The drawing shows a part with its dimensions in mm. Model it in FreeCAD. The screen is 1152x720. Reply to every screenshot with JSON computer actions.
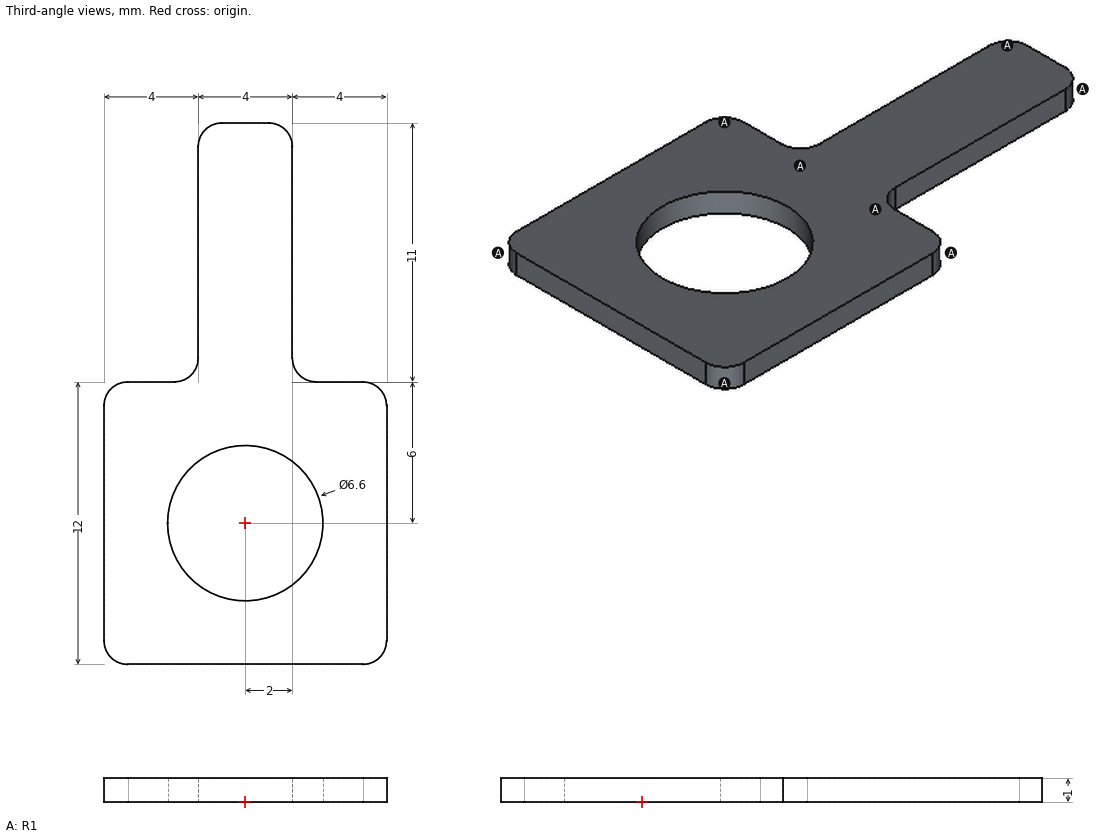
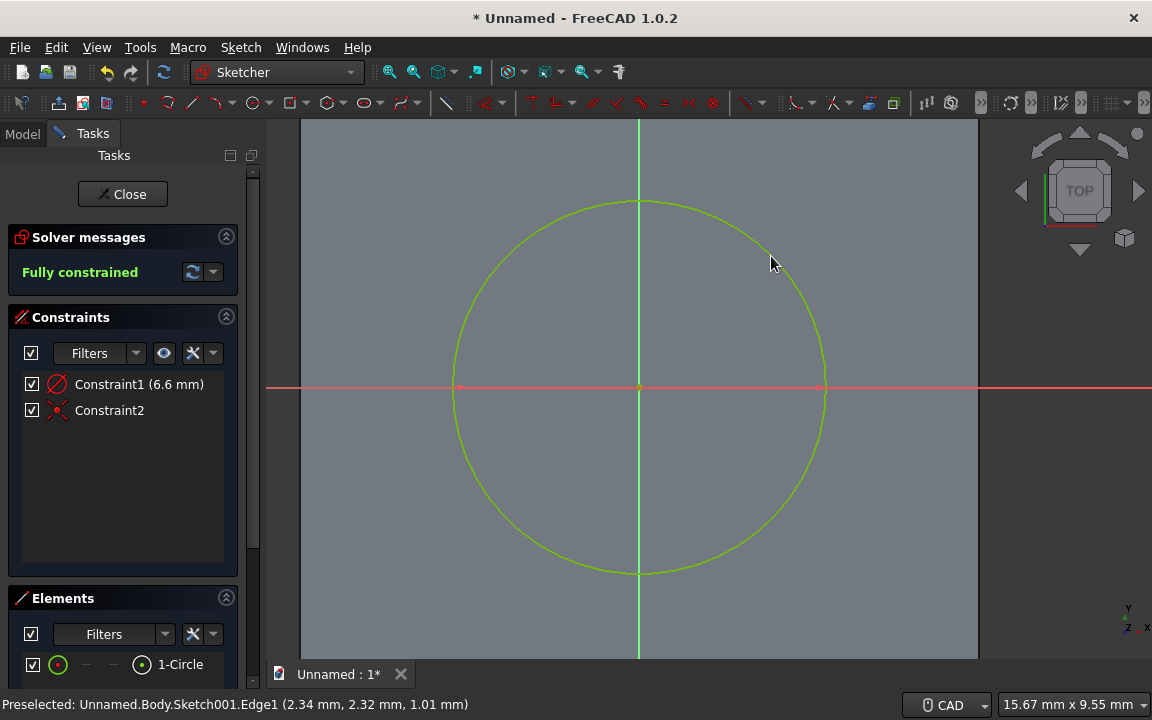
{"action": "left_click", "coordinate": [123, 194]}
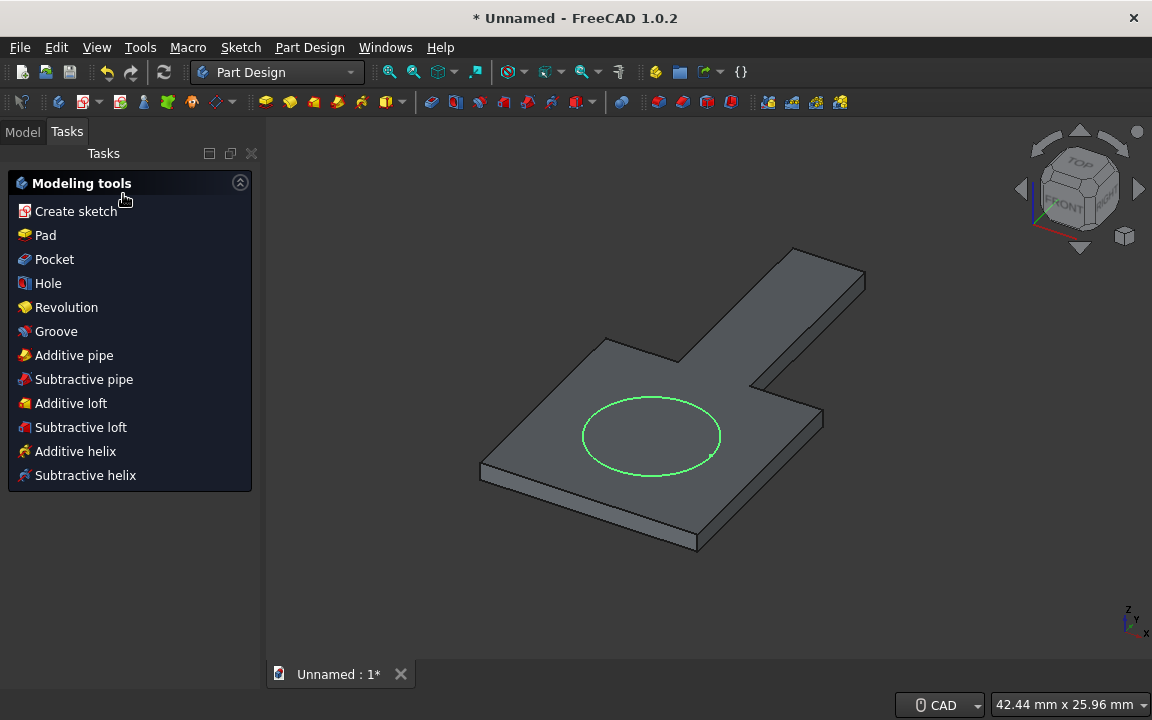
{"action": "left_click", "coordinate": [432, 102]}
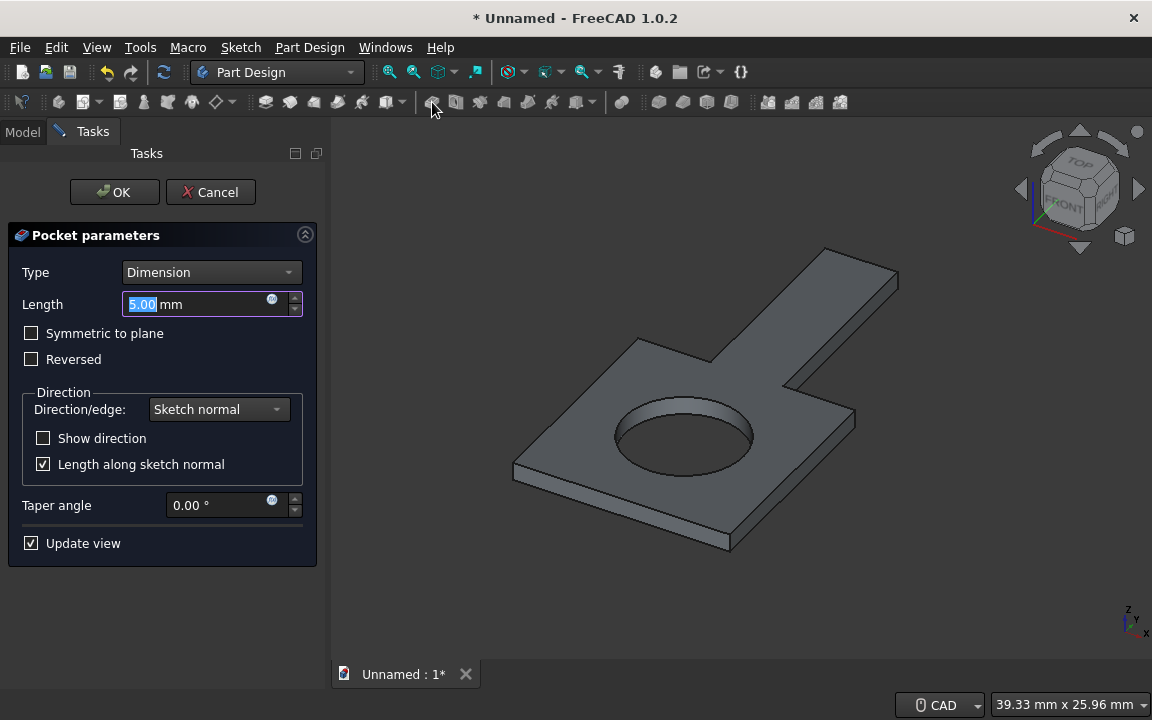
{"action": "left_click", "coordinate": [212, 272]}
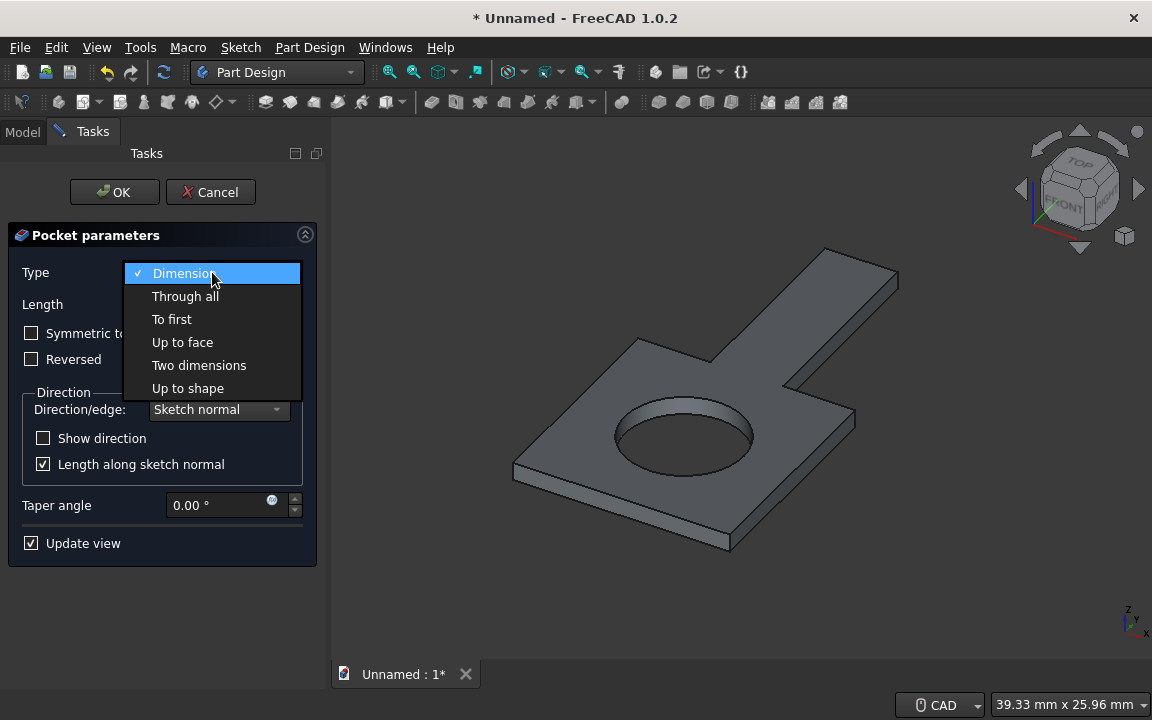
{"action": "left_click", "coordinate": [212, 296]}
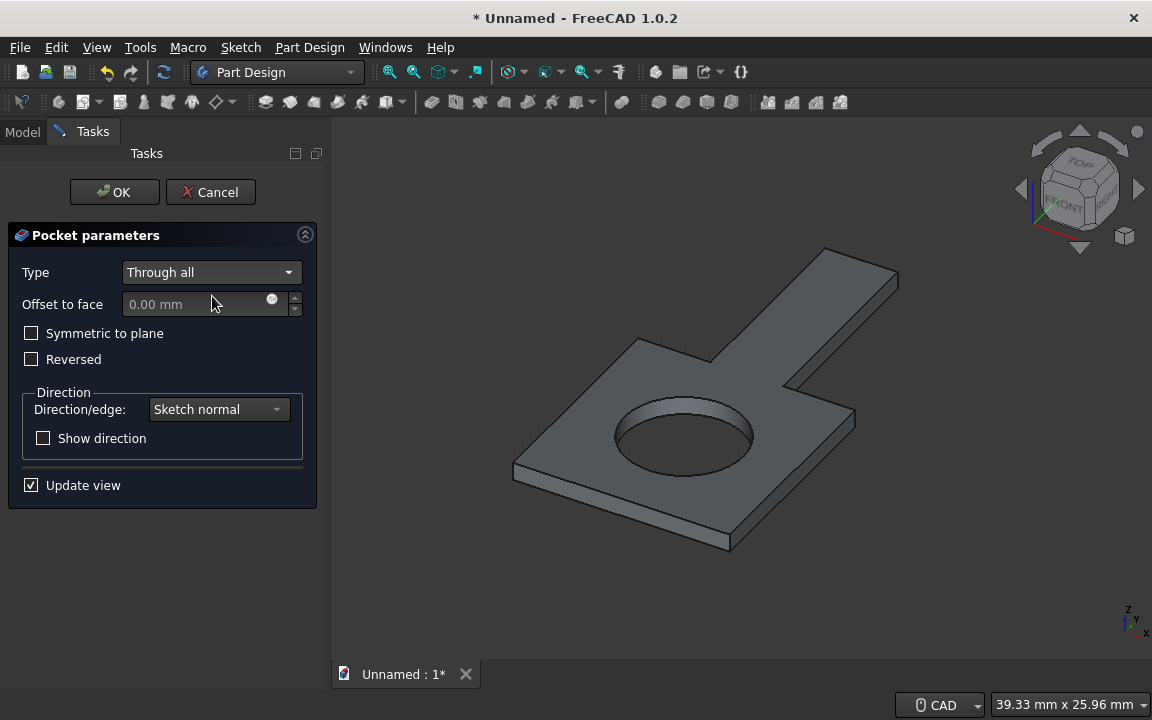
{"action": "left_click", "coordinate": [115, 192]}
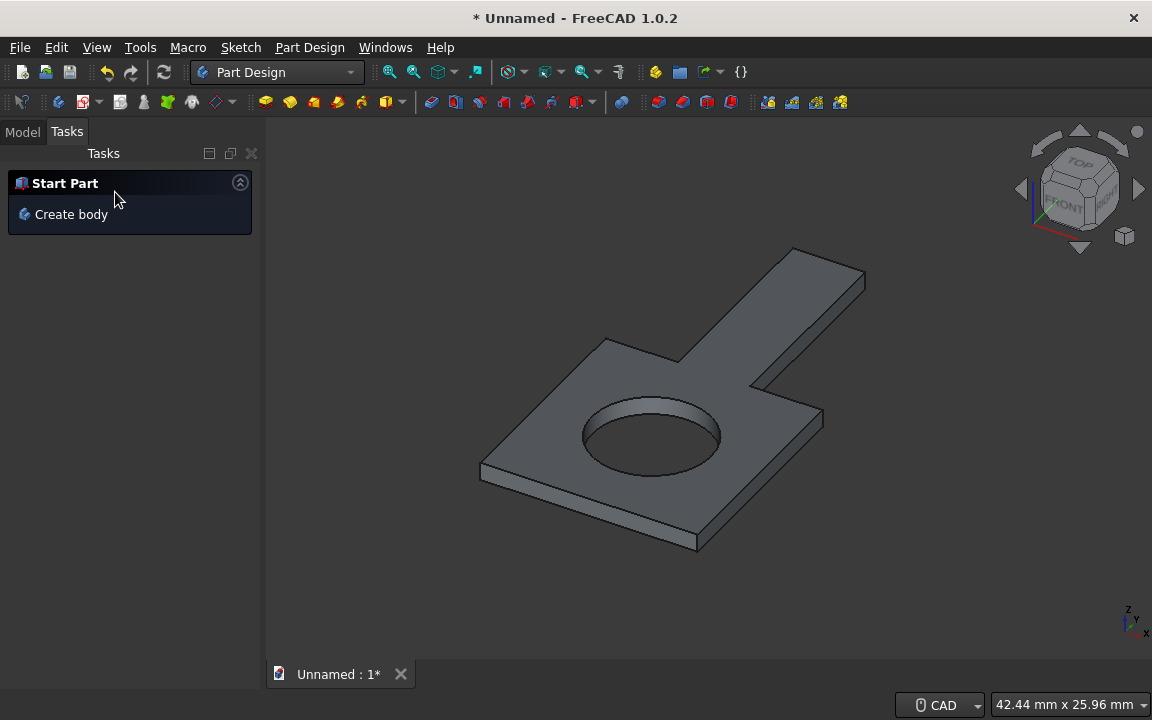
{"action": "left_click", "coordinate": [697, 542]}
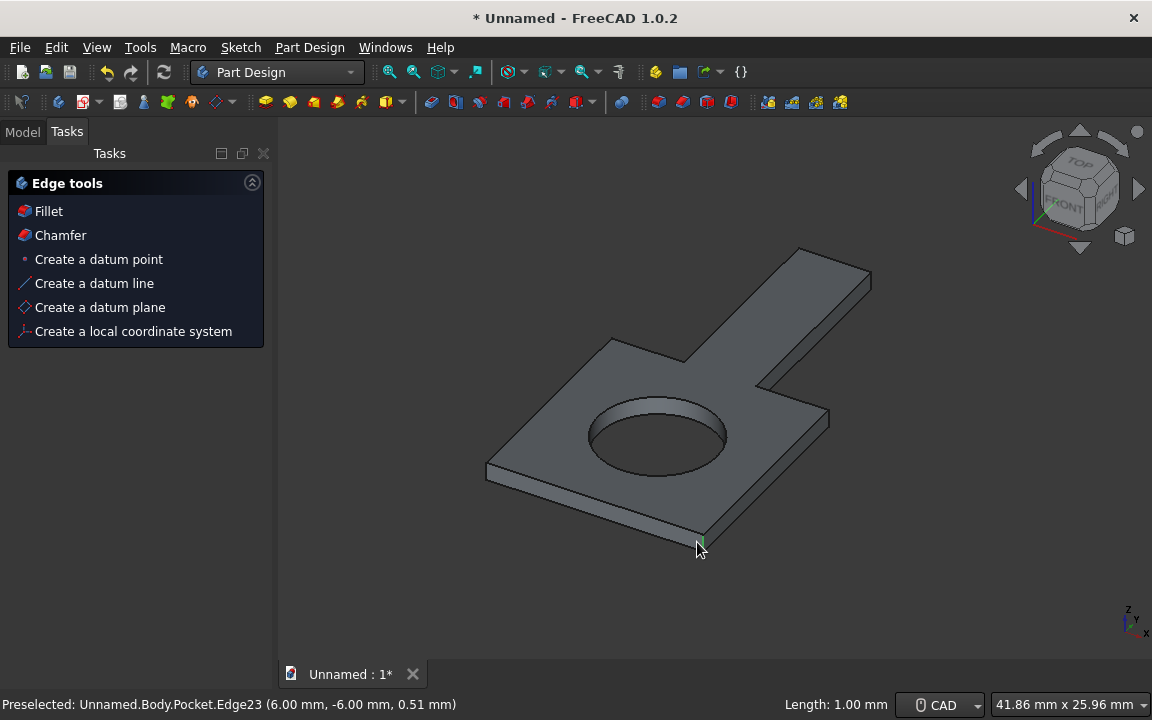
{"action": "scroll", "coordinate": [486, 470], "scroll_direction": "up", "scroll_amount": 4}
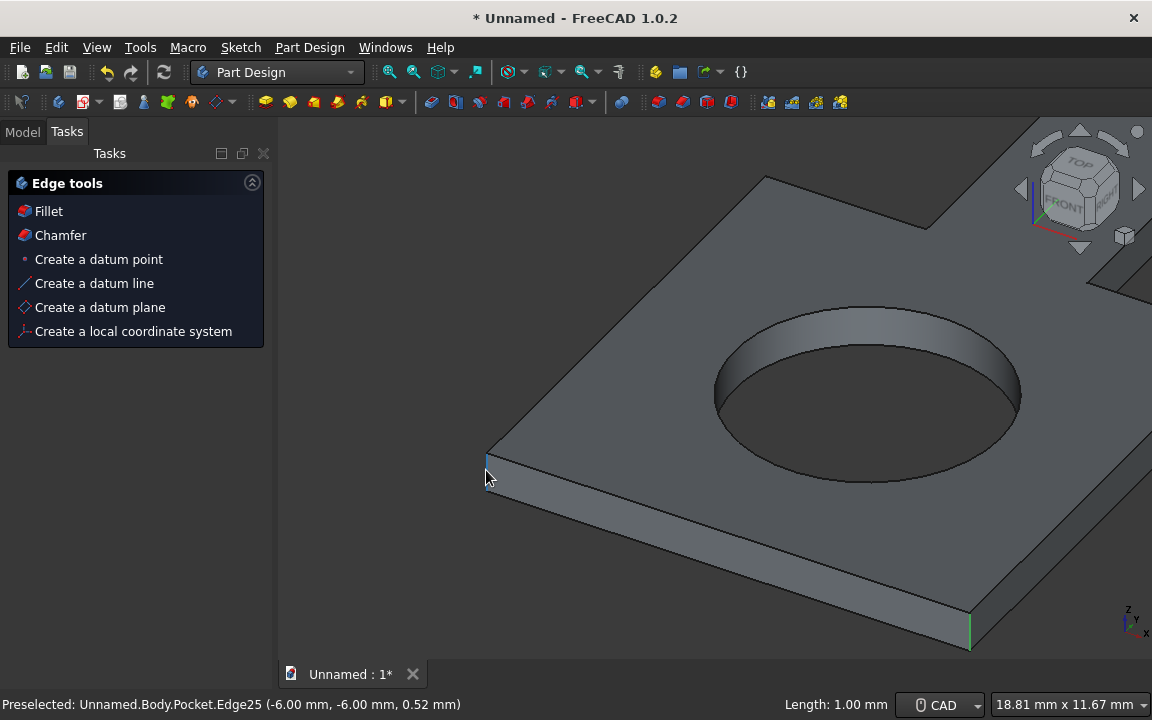
{"action": "left_click", "coordinate": [390, 72]}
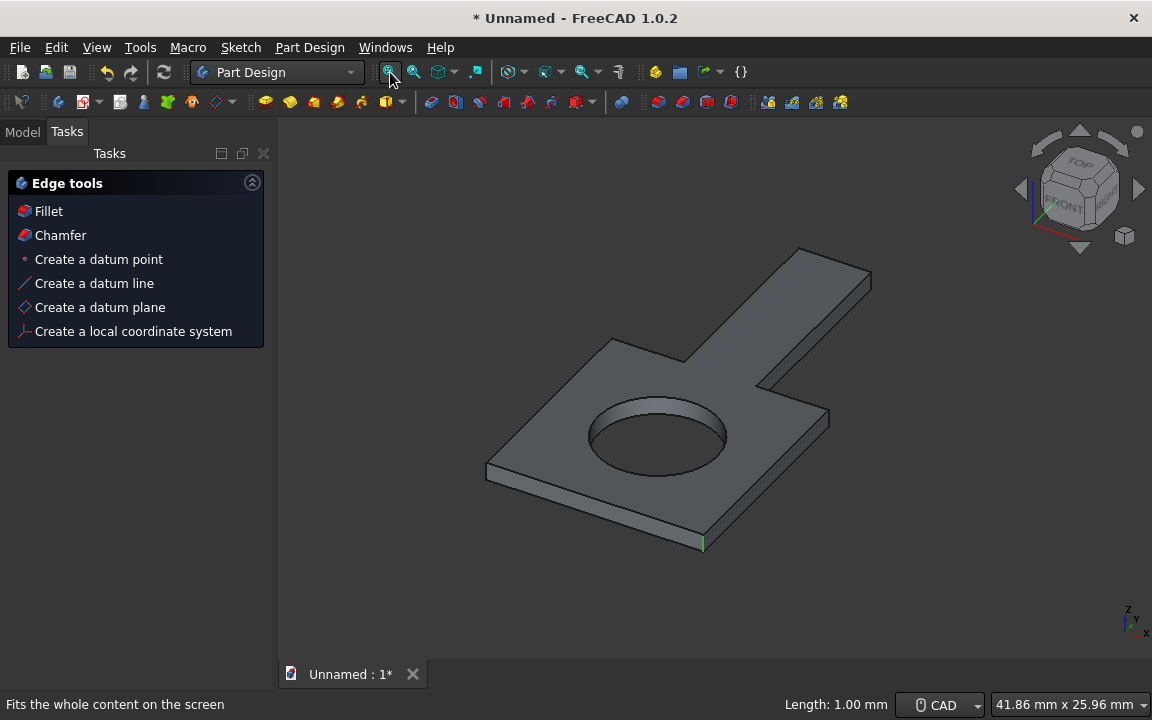
{"action": "key", "text": "0"}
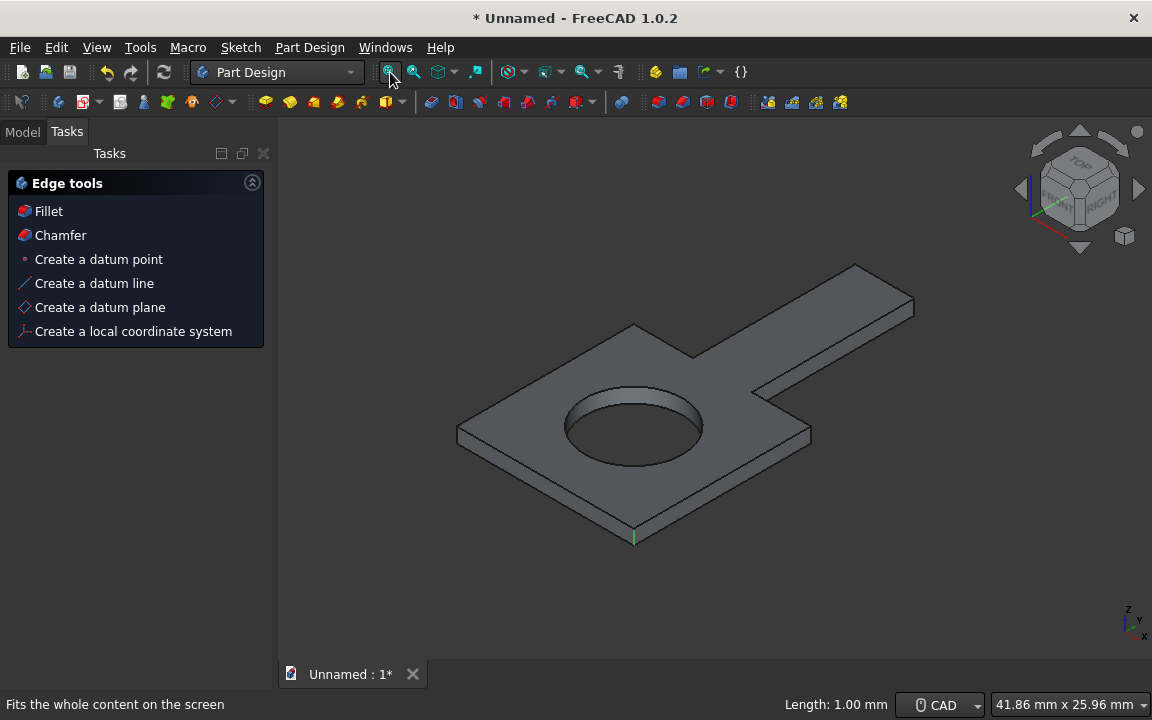
{"action": "scroll", "coordinate": [457, 434], "scroll_direction": "up", "scroll_amount": 4}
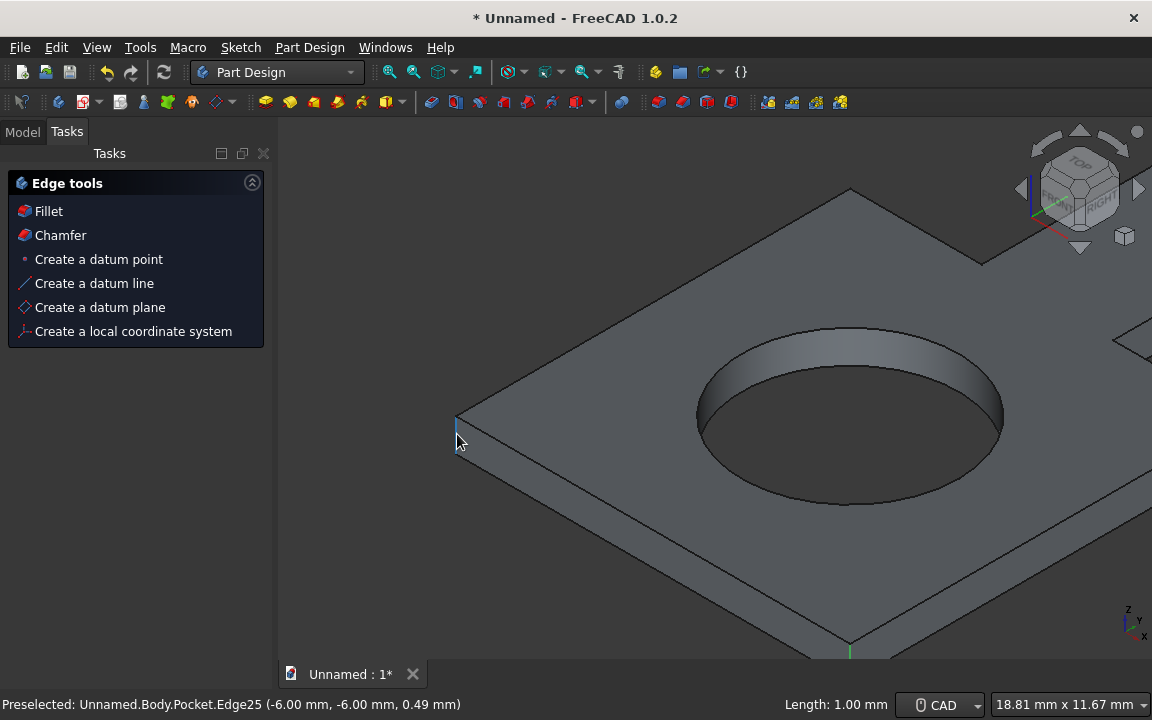
{"action": "key", "text": "v f"}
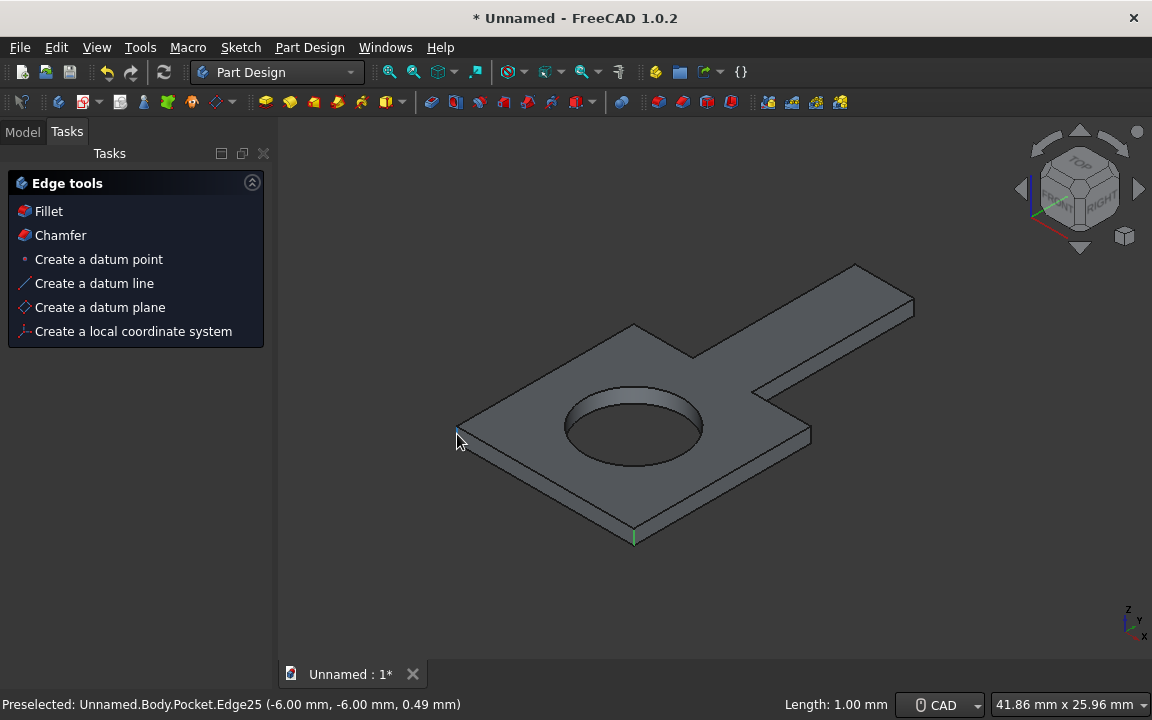
{"action": "key", "text": "2"}